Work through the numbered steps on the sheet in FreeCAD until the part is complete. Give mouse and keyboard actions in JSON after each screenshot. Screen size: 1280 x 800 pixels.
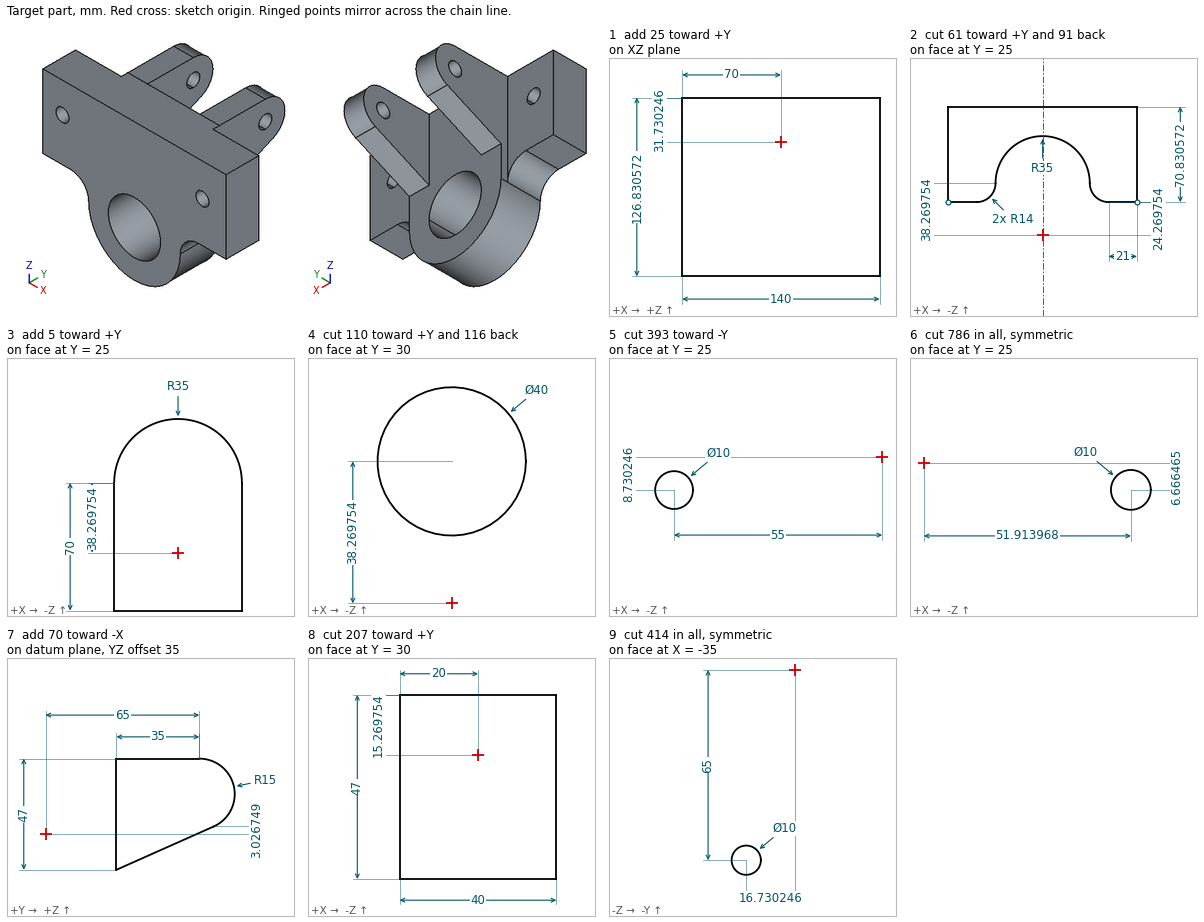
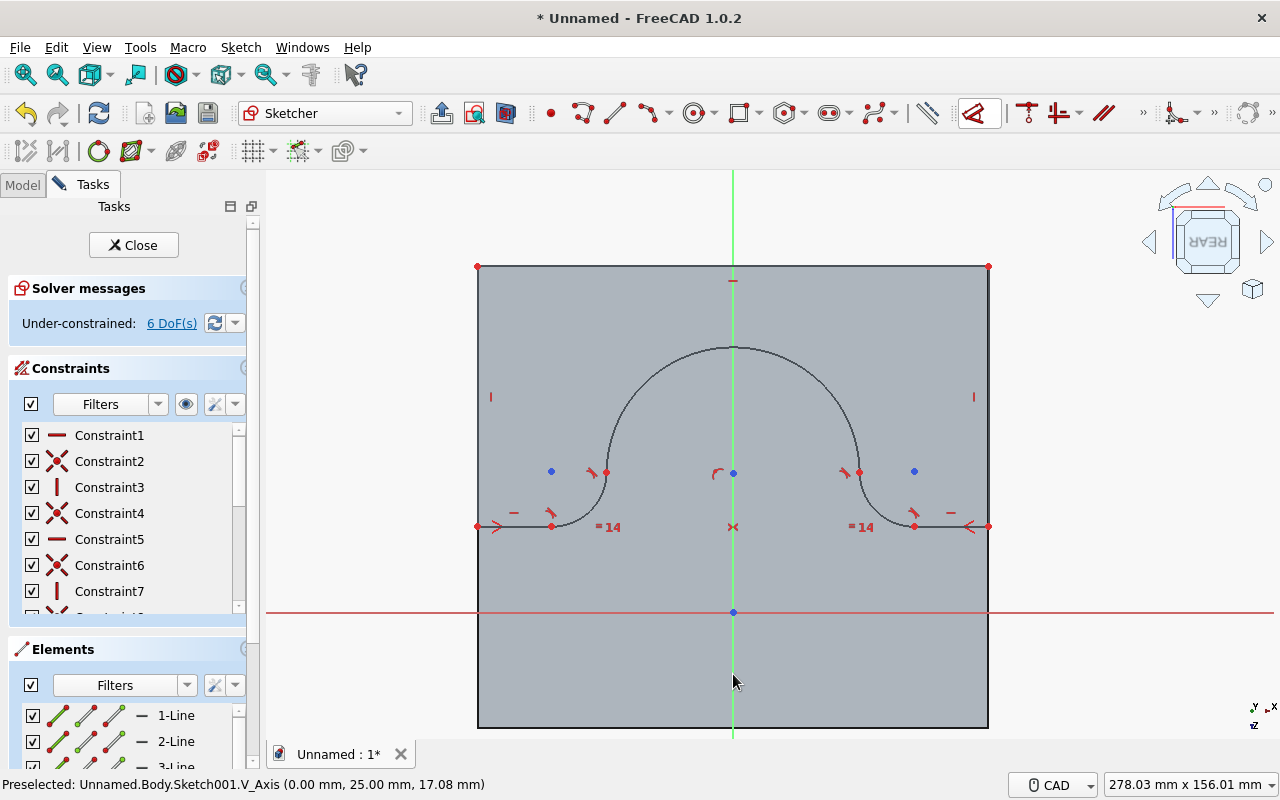
{"action": "left_click", "coordinate": [577, 521]}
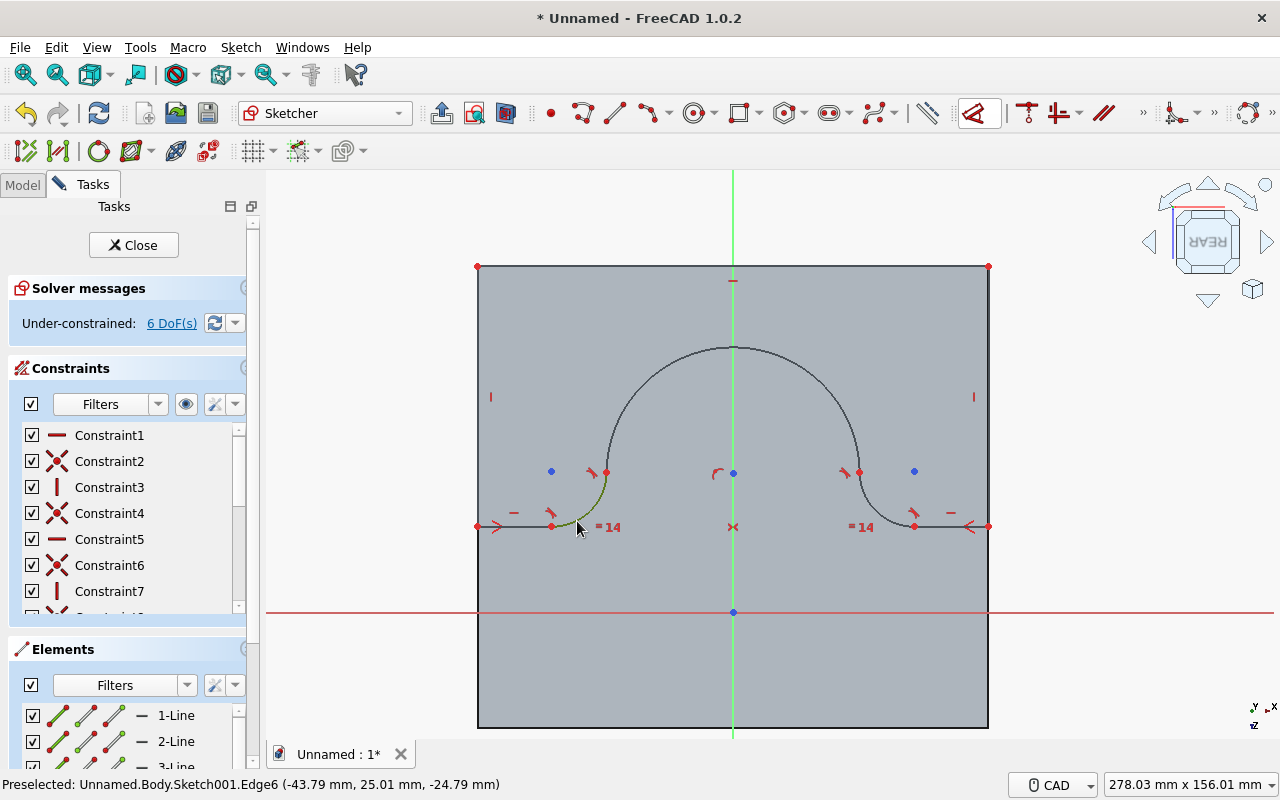
{"action": "left_click", "coordinate": [996, 114]}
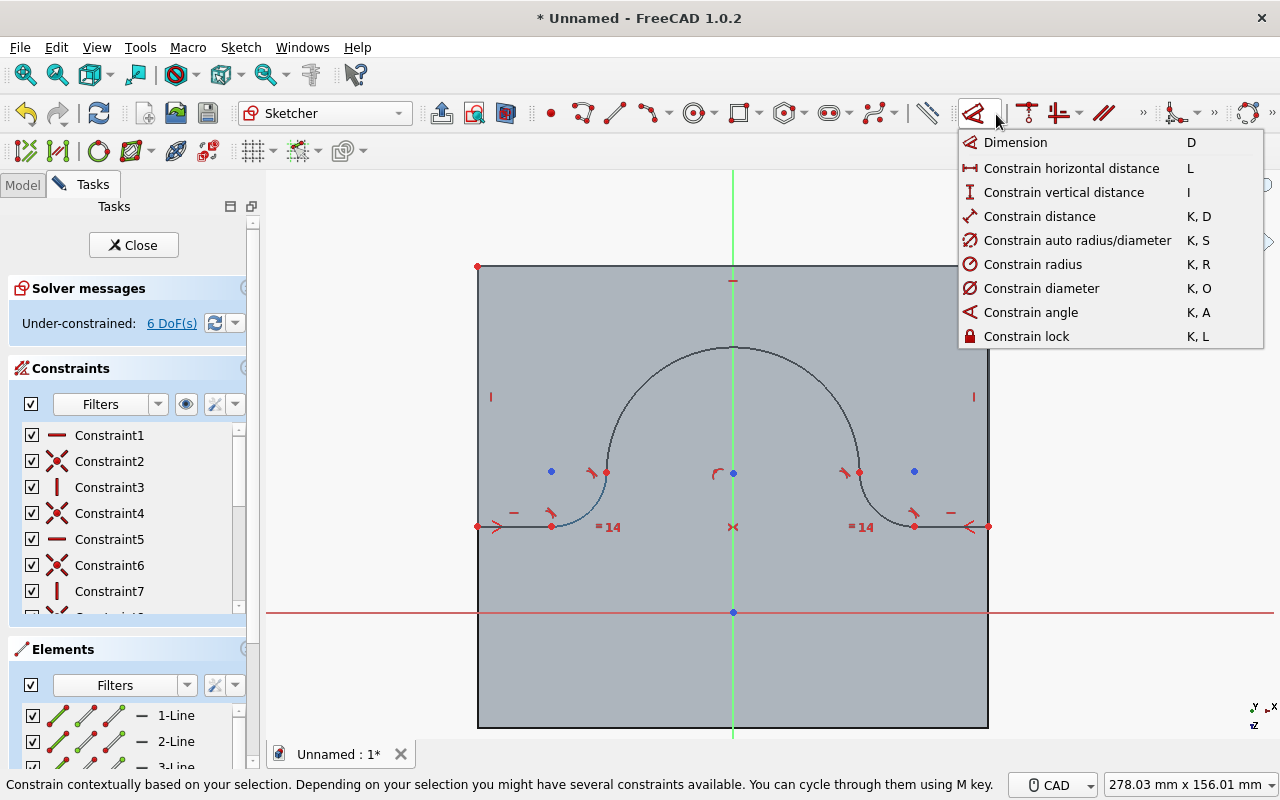
{"action": "left_click", "coordinate": [1111, 264]}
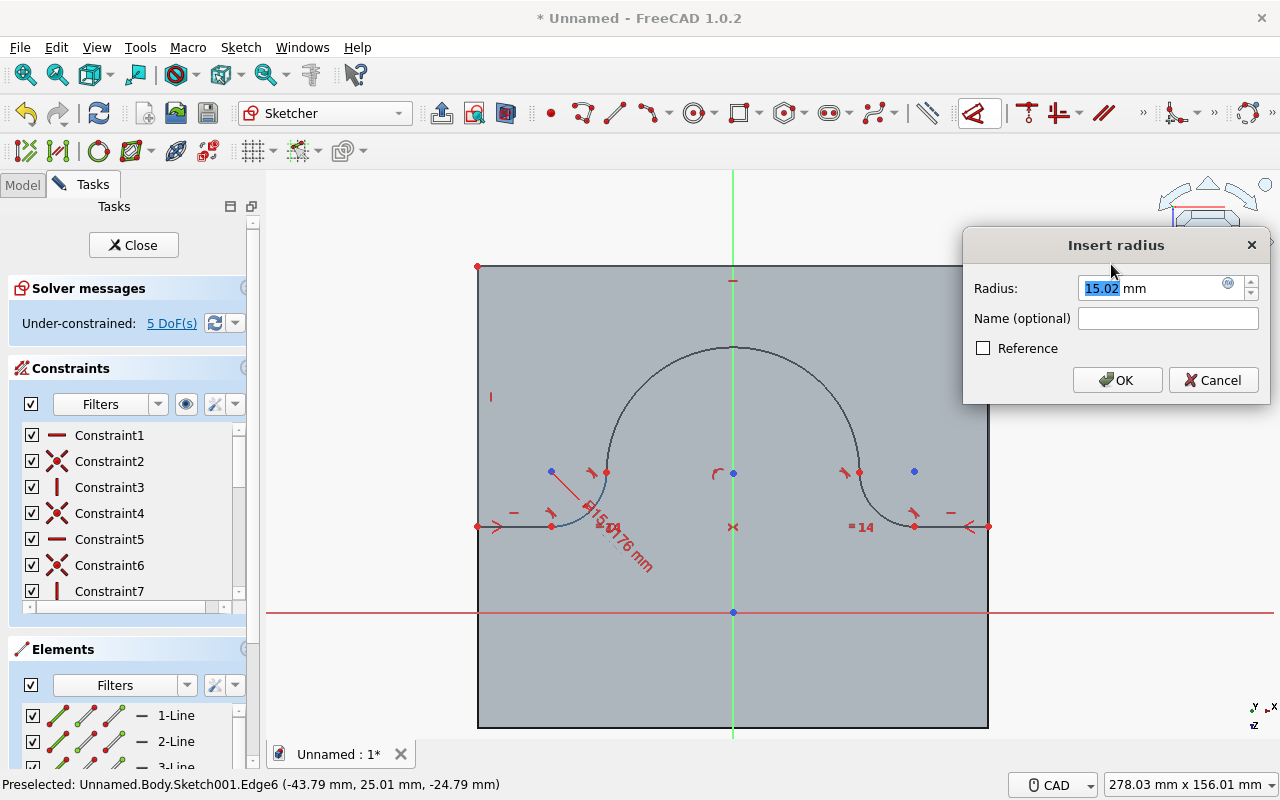
{"action": "type", "text": "14"}
{"action": "key", "text": "Return"}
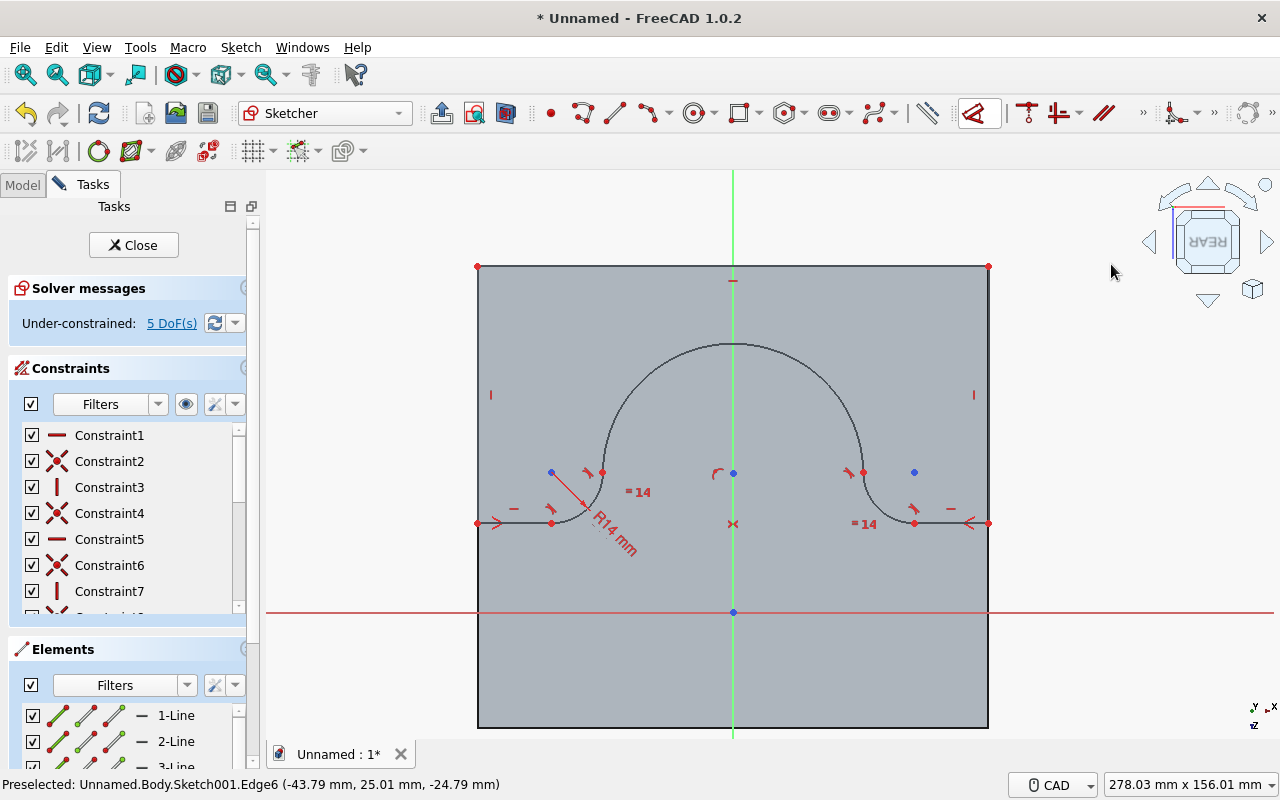
{"action": "left_click", "coordinate": [809, 368]}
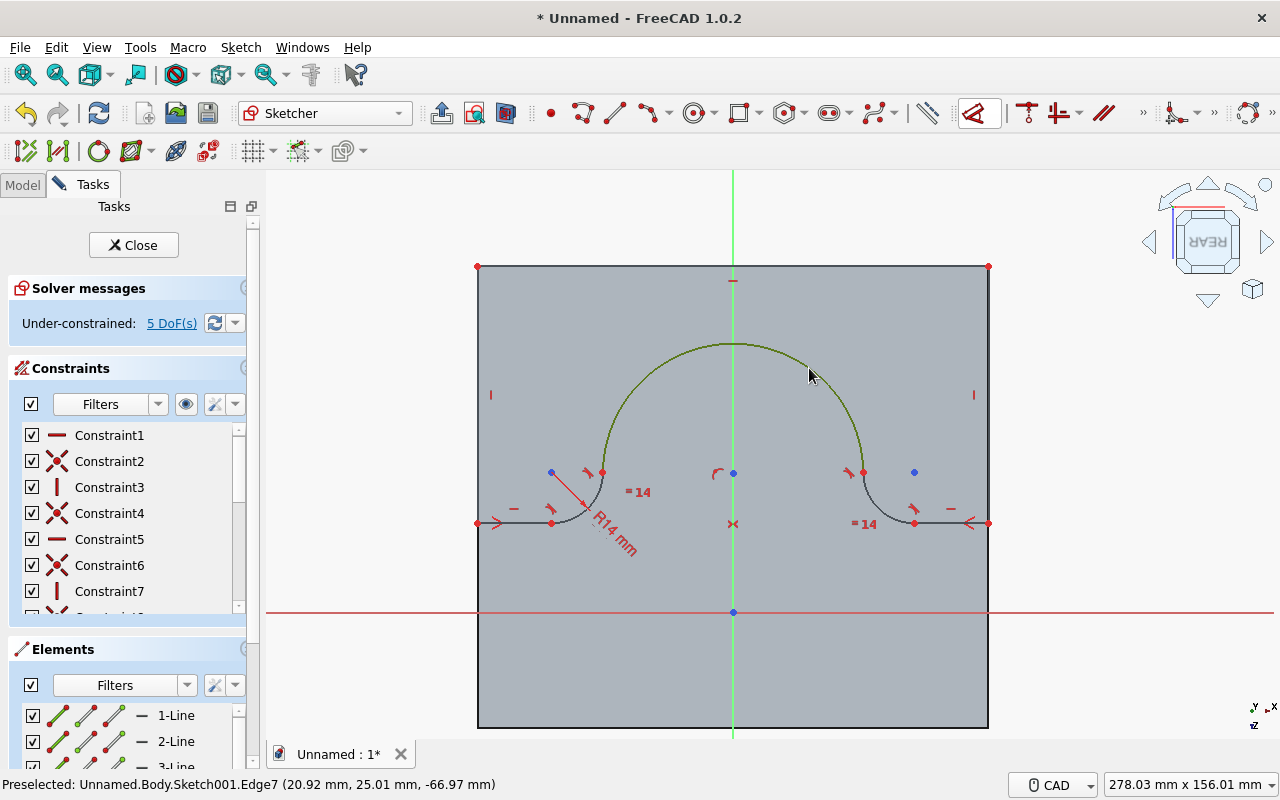
{"action": "key", "text": "k r"}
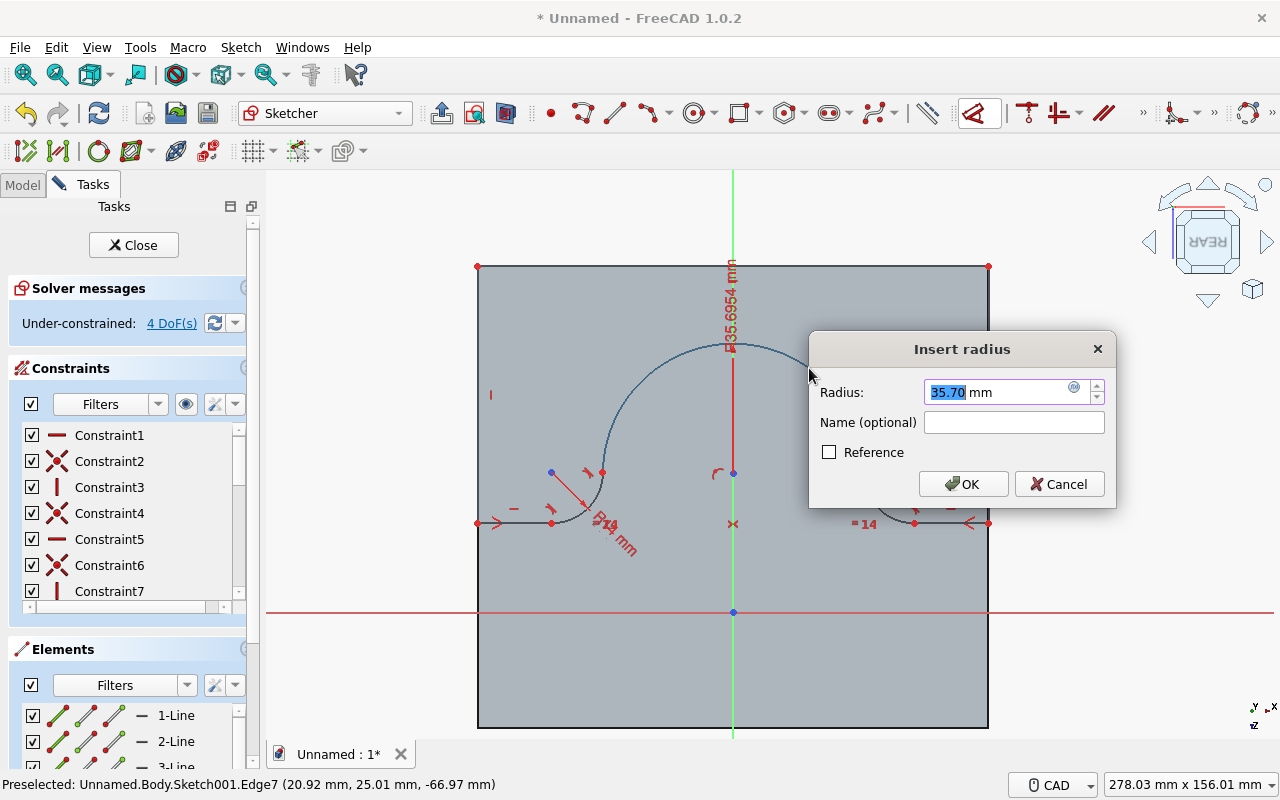
{"action": "type", "text": "35"}
{"action": "key", "text": "Return"}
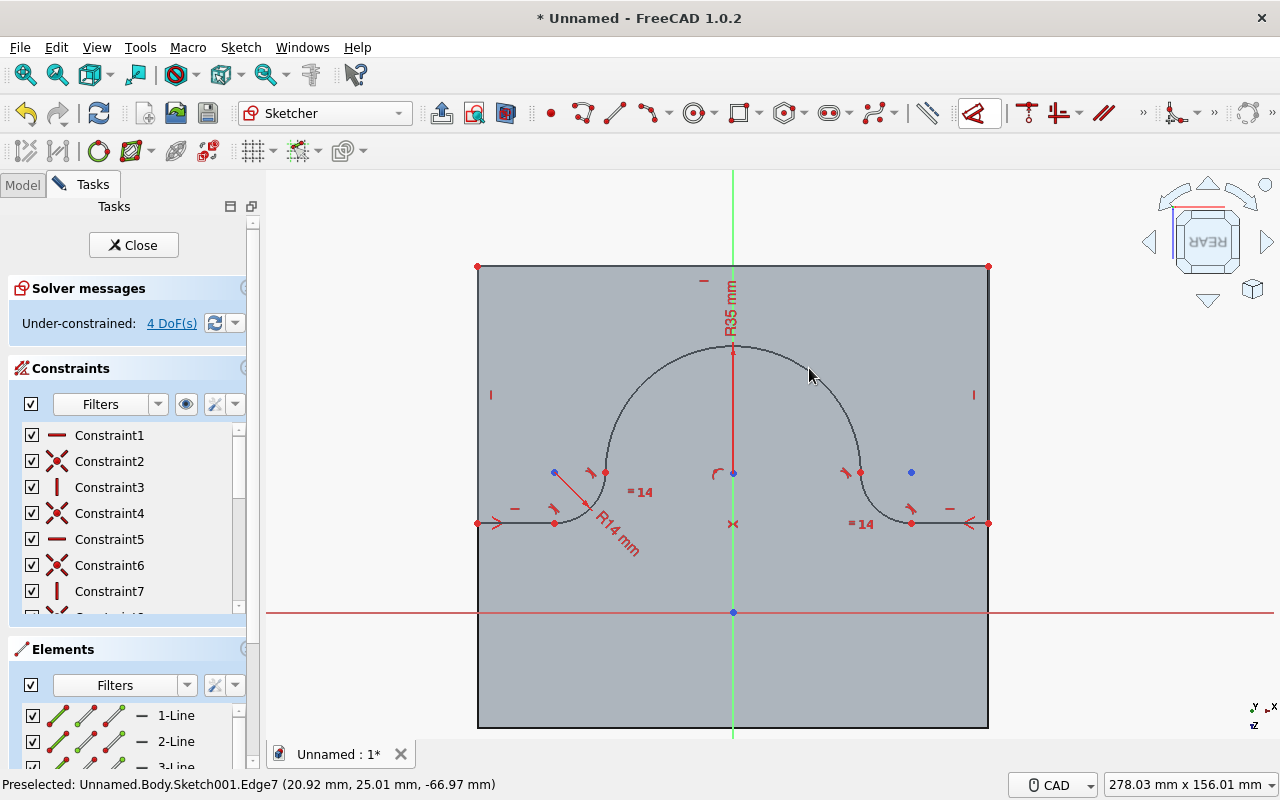
{"action": "left_click", "coordinate": [935, 523]}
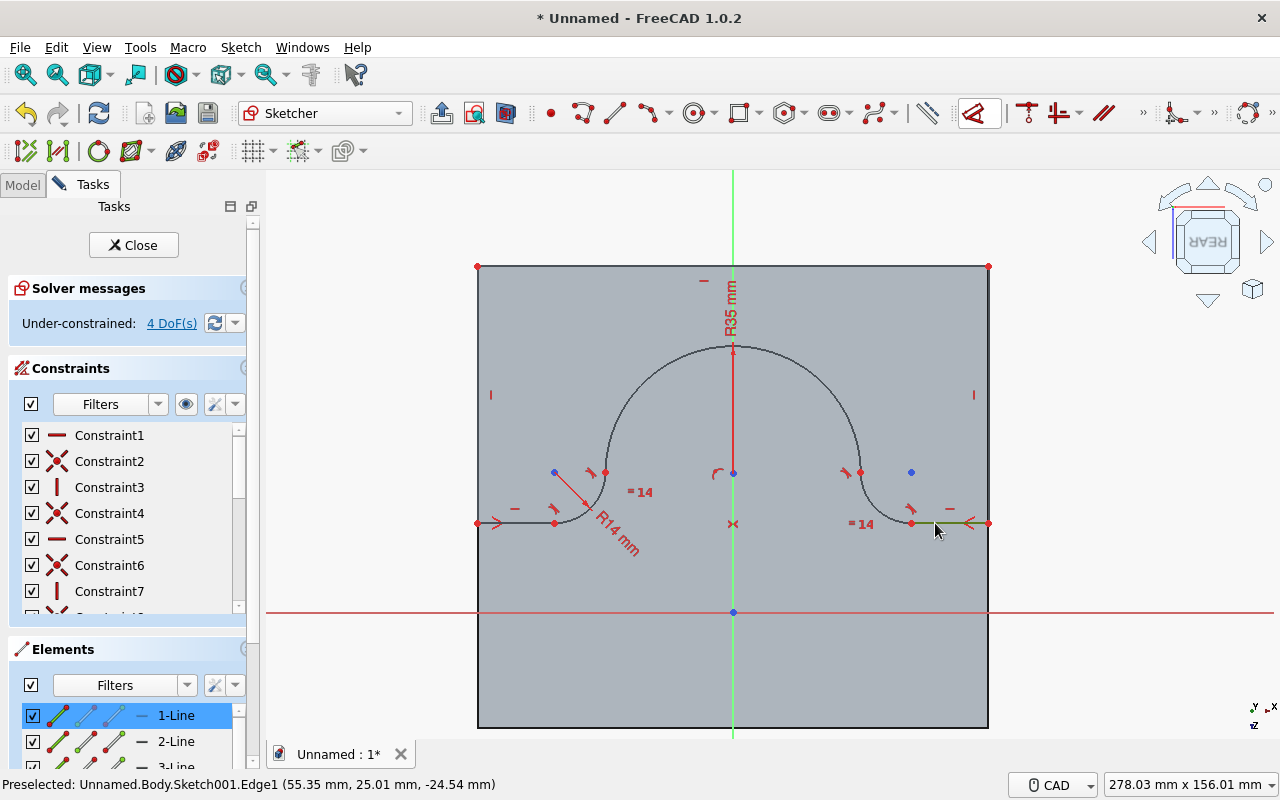
{"action": "left_click", "coordinate": [996, 114]}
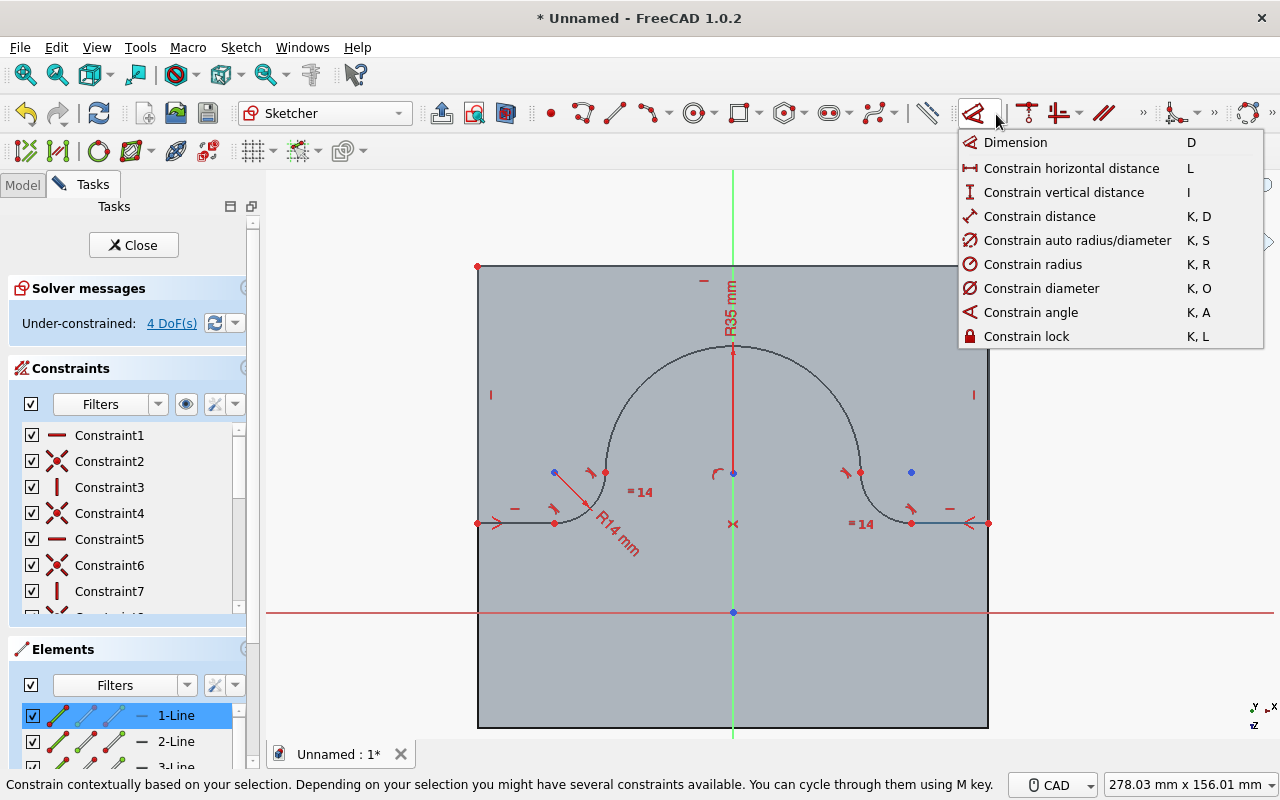
{"action": "left_click", "coordinate": [1111, 168]}